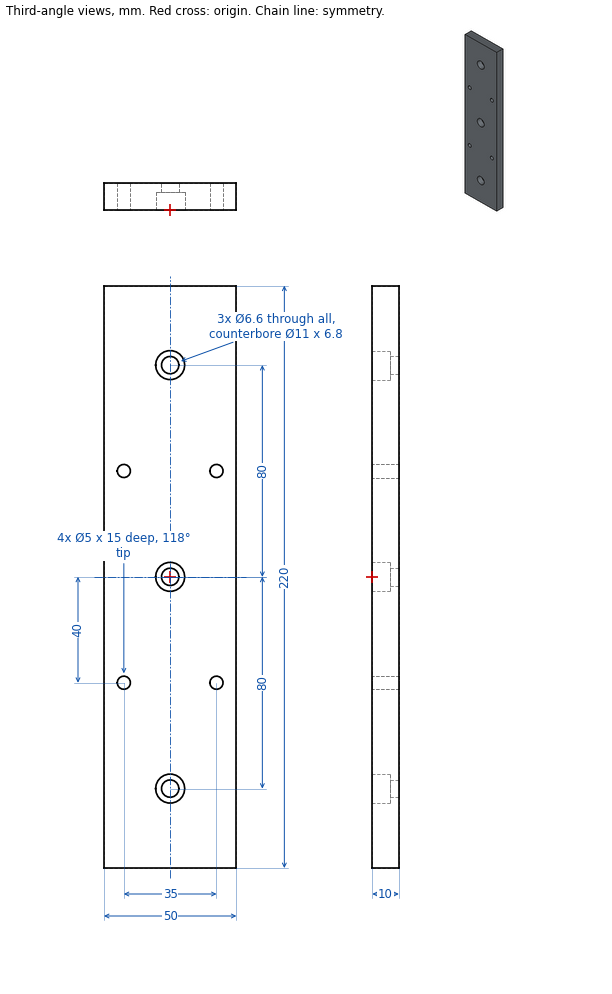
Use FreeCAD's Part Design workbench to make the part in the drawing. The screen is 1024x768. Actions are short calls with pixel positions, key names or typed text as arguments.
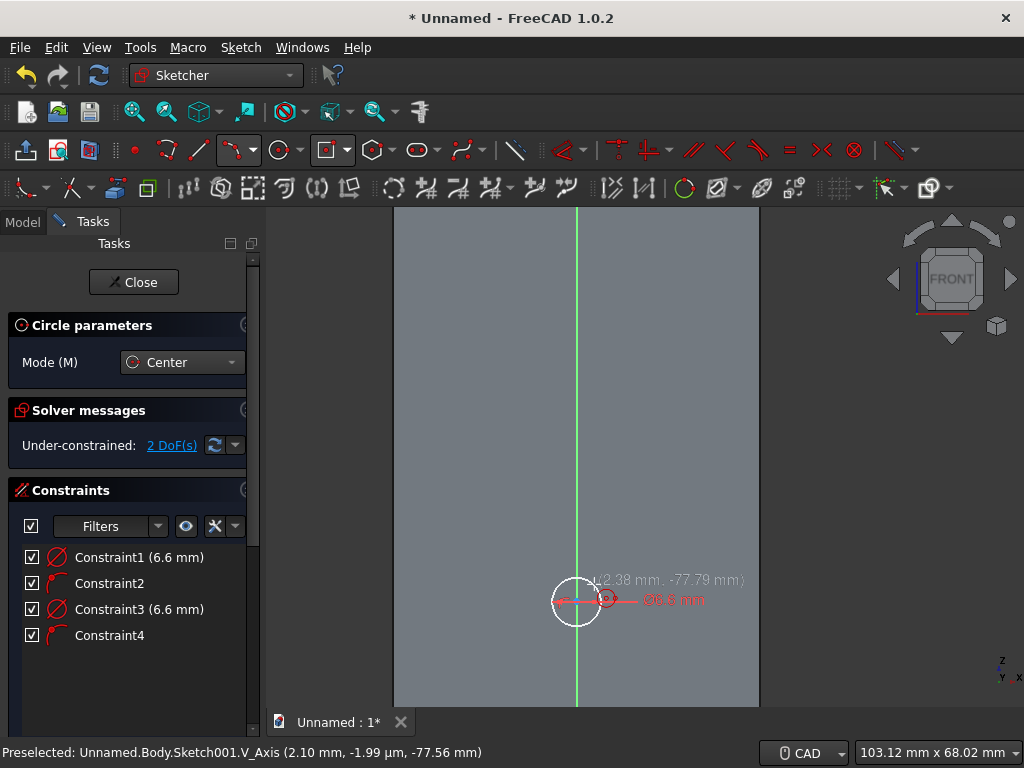
scroll(576, 602, down, 7)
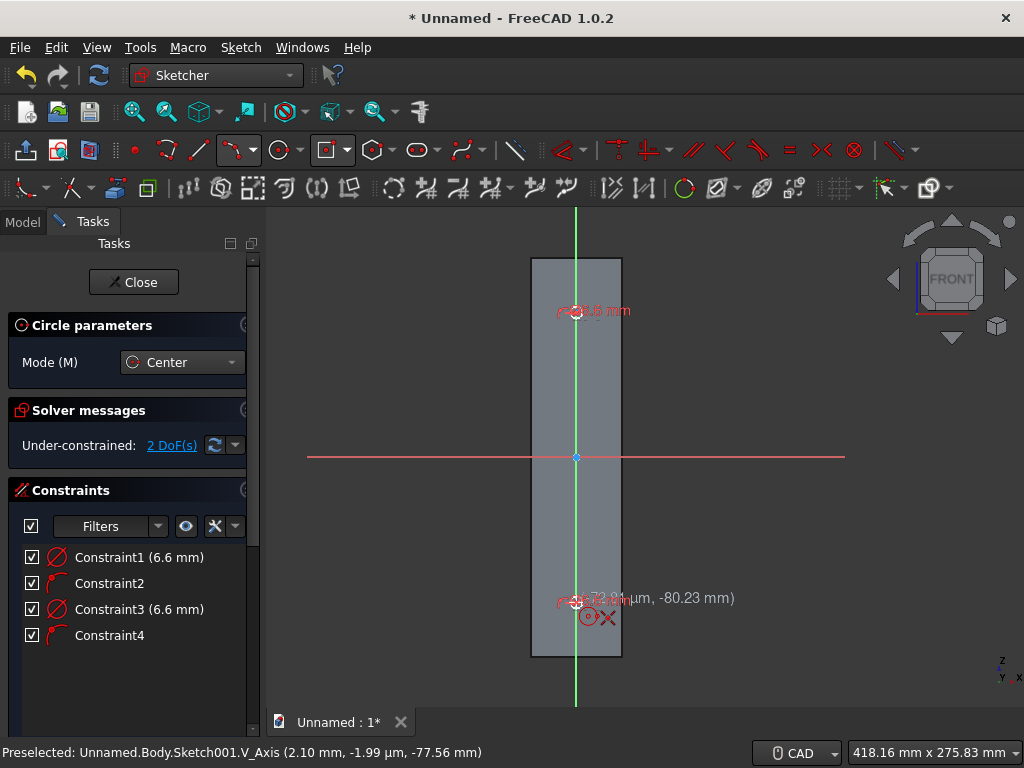
scroll(576, 457, up, 7)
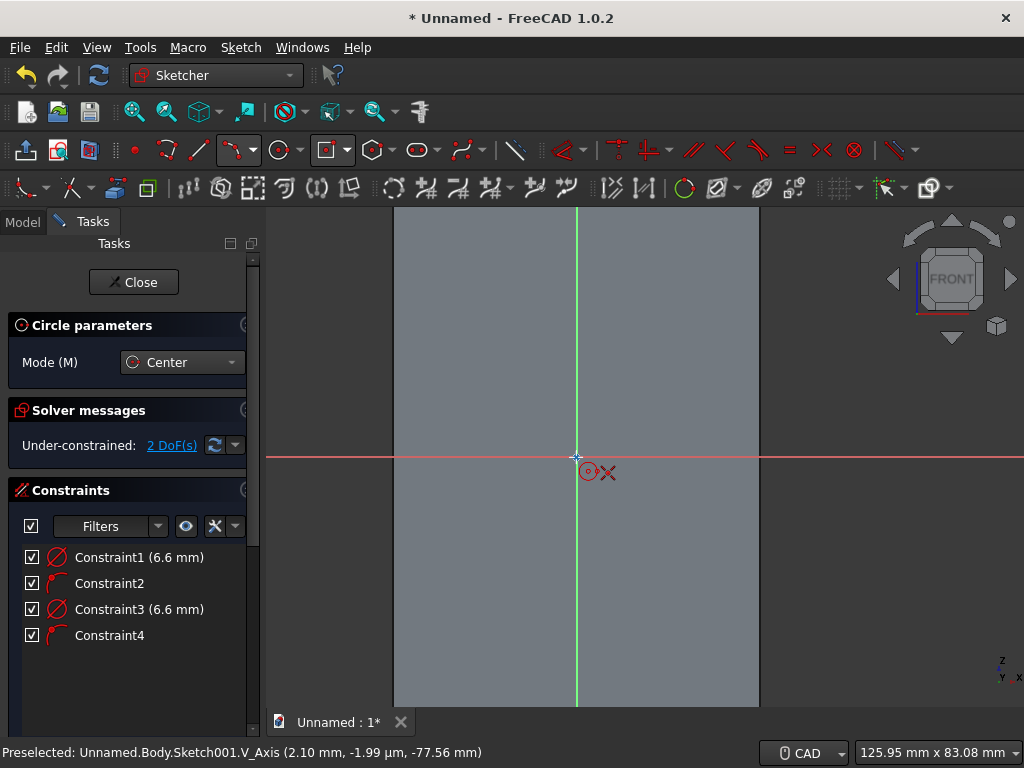
click(577, 457)
move(594, 440)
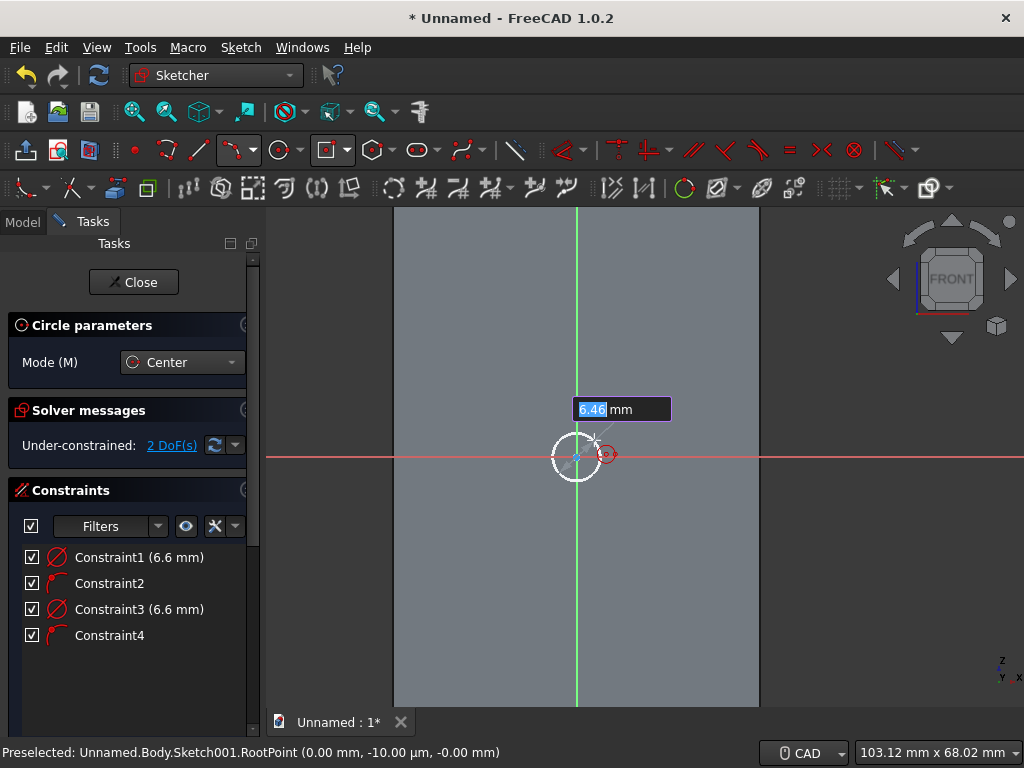
text(6.6)
key(Return)
key(Escape)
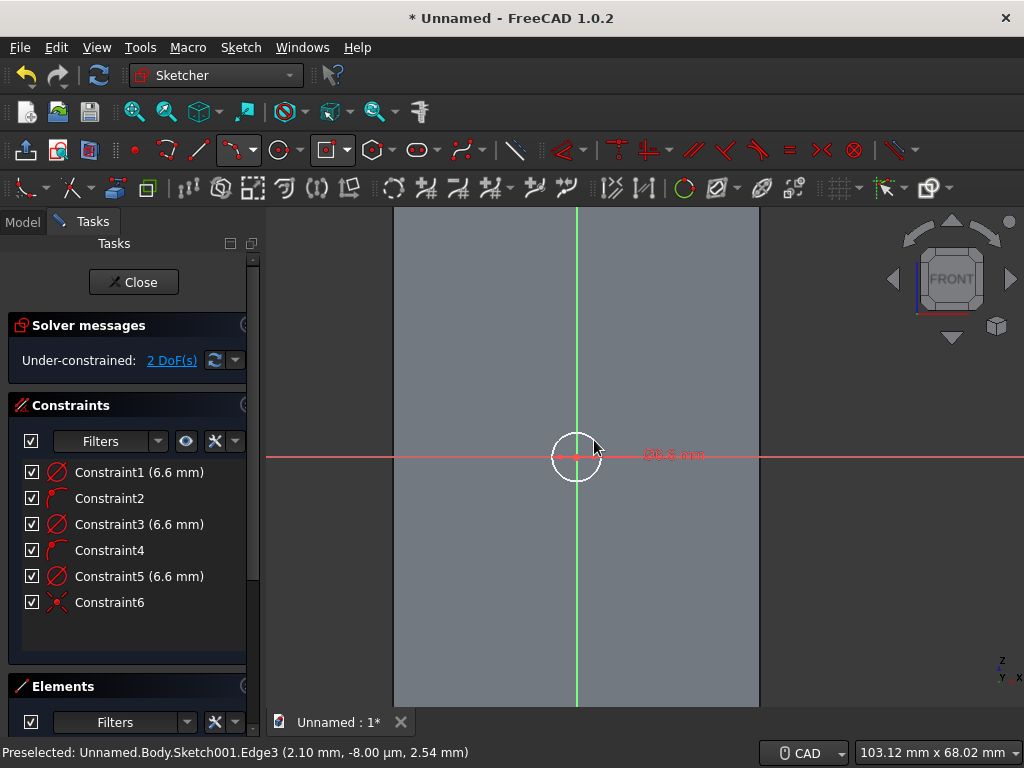
click(562, 150)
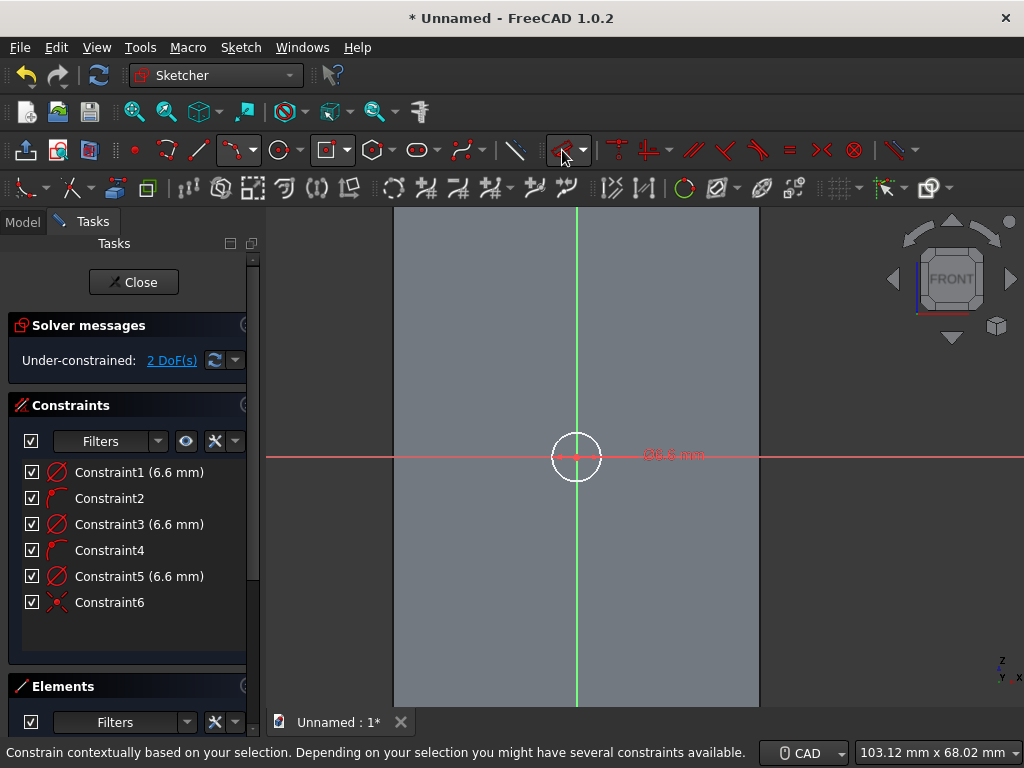
scroll(576, 457, down, 7)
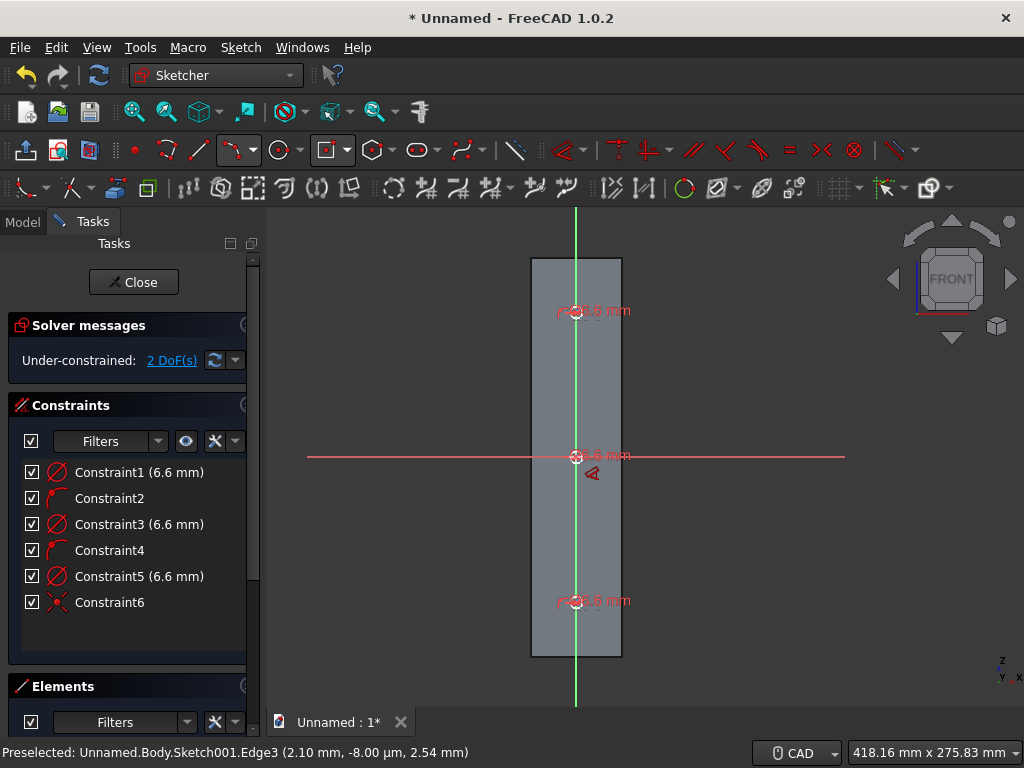
click(576, 313)
click(610, 385)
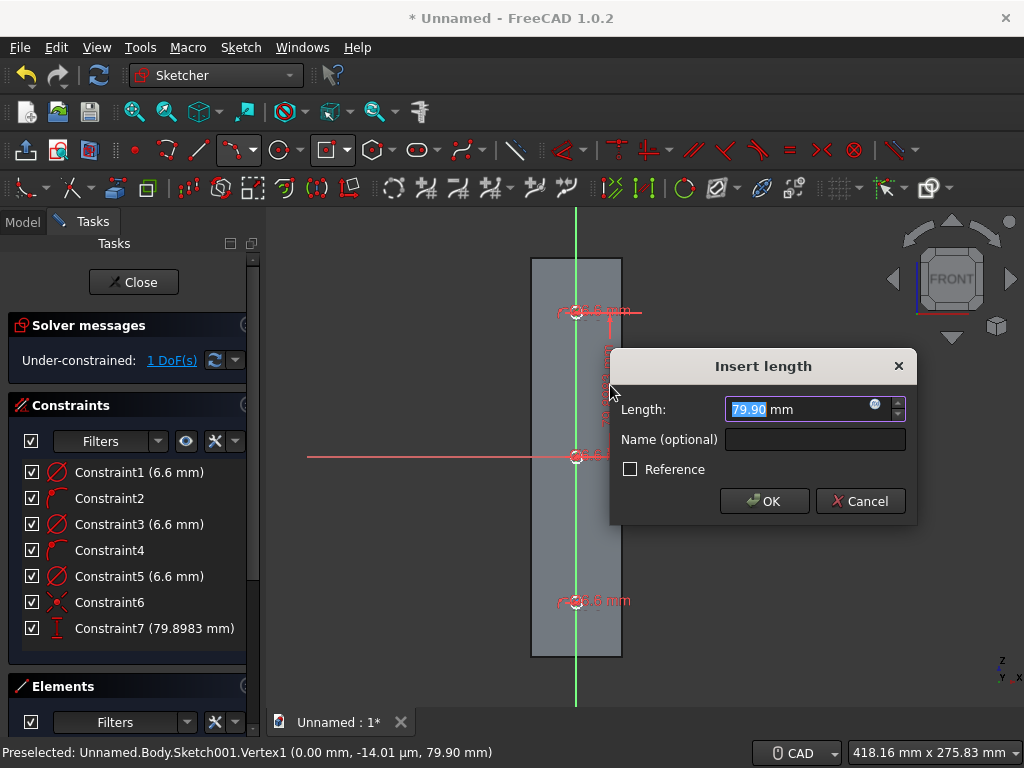
text(80)
key(Return)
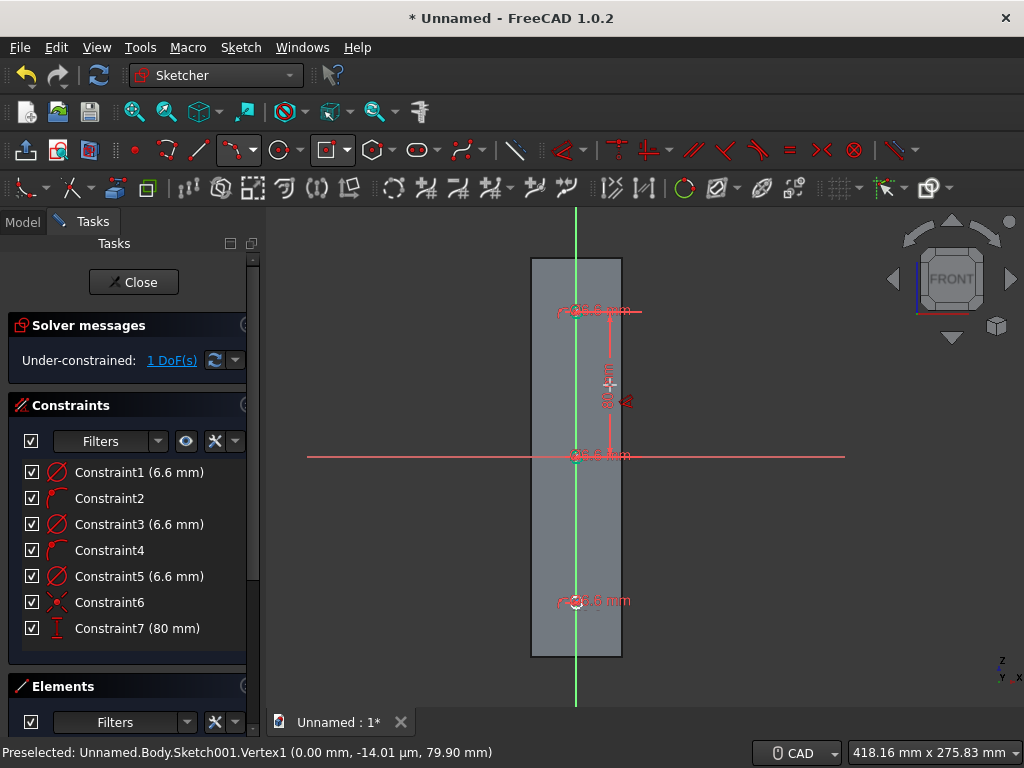
click(576, 603)
click(610, 530)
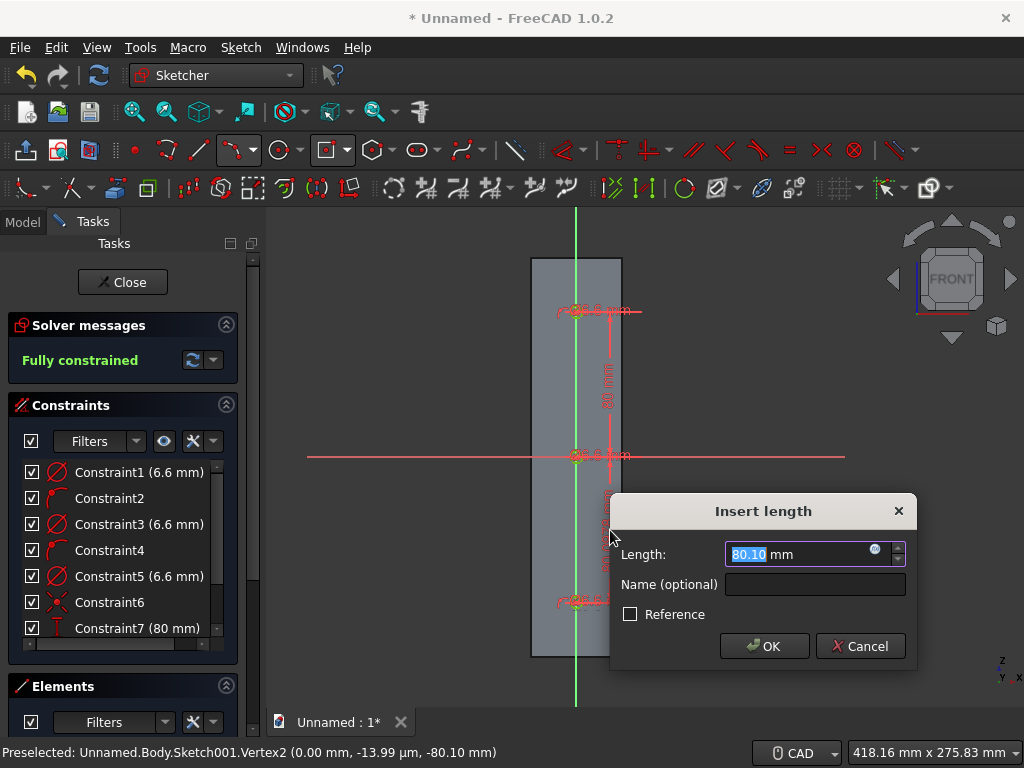
text(80)
key(Return)
key(Escape)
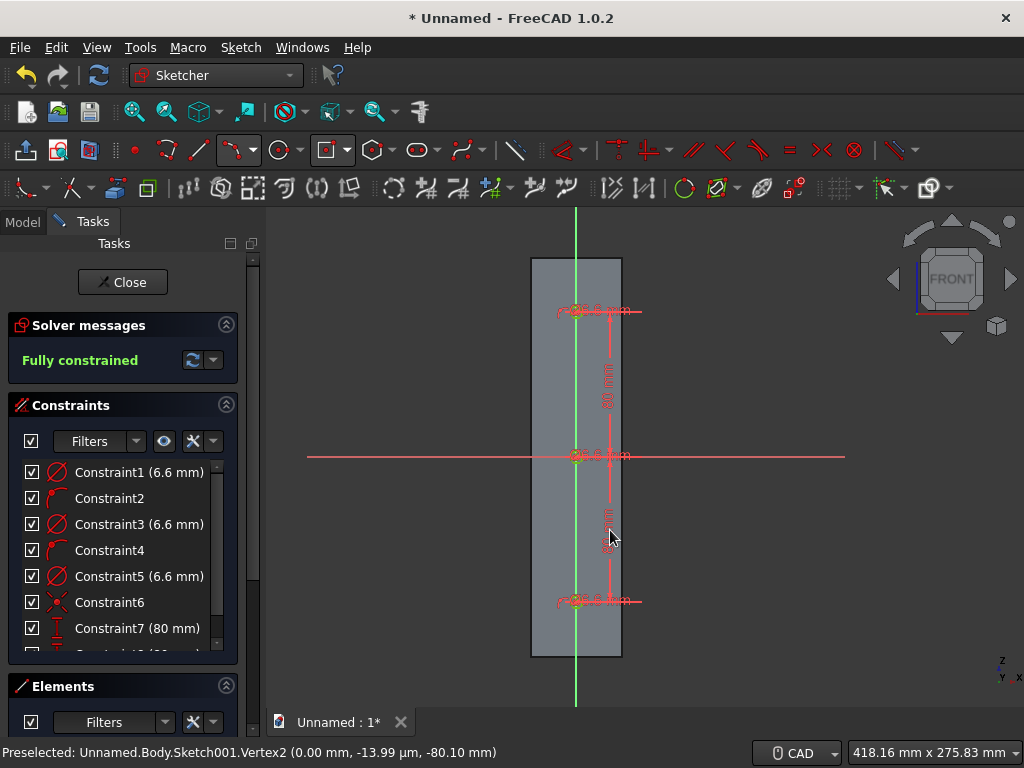
click(123, 282)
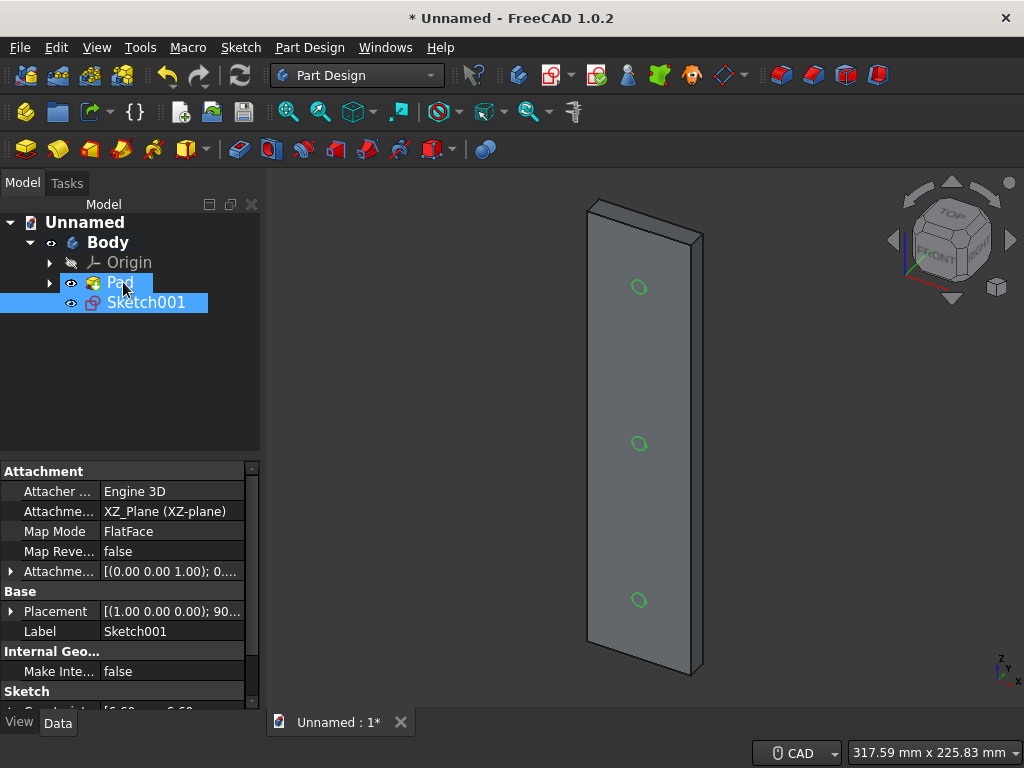
click(272, 150)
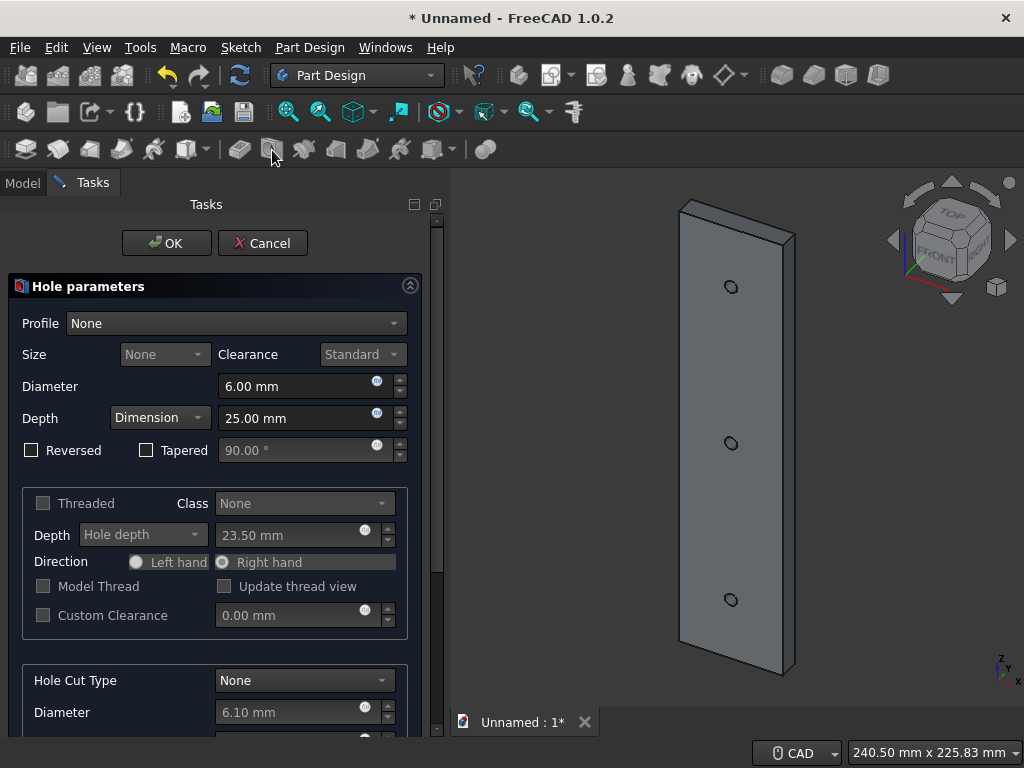
triple_click(305, 386)